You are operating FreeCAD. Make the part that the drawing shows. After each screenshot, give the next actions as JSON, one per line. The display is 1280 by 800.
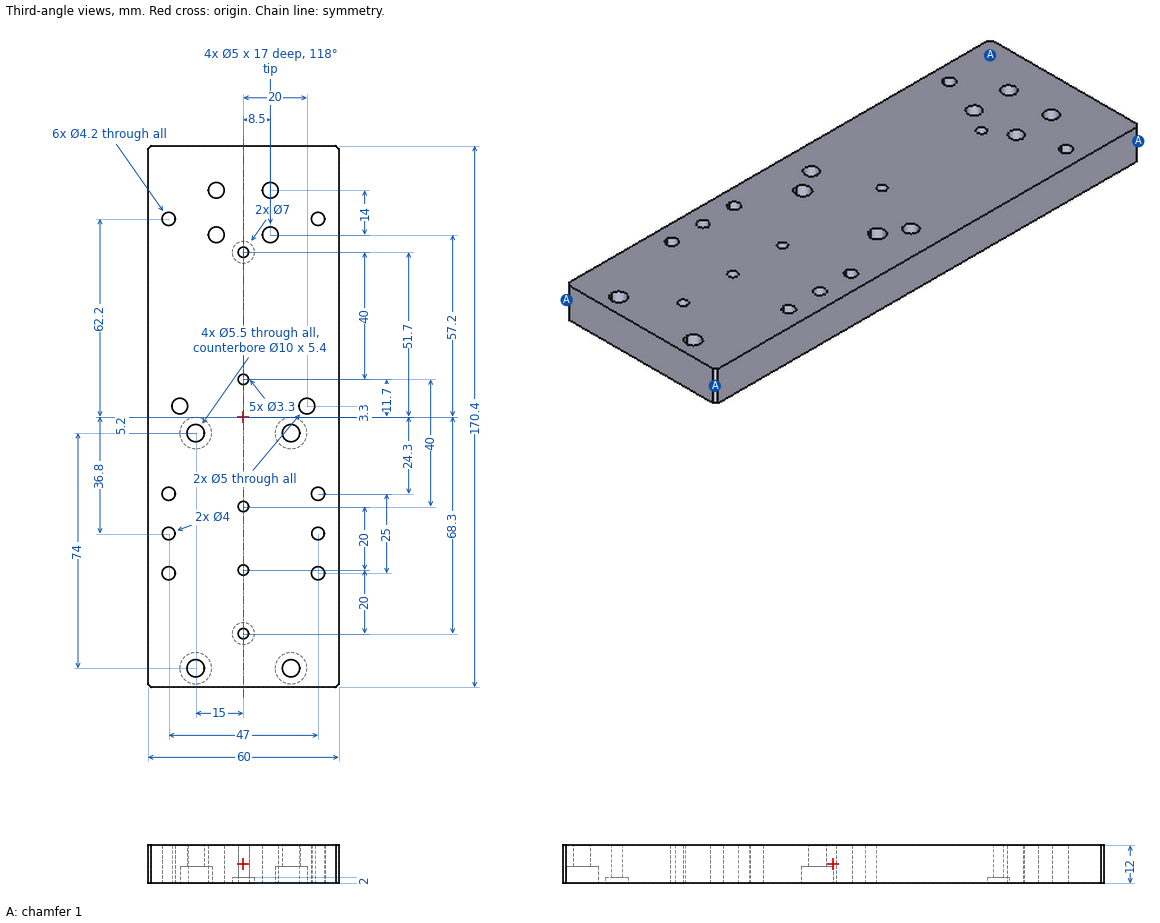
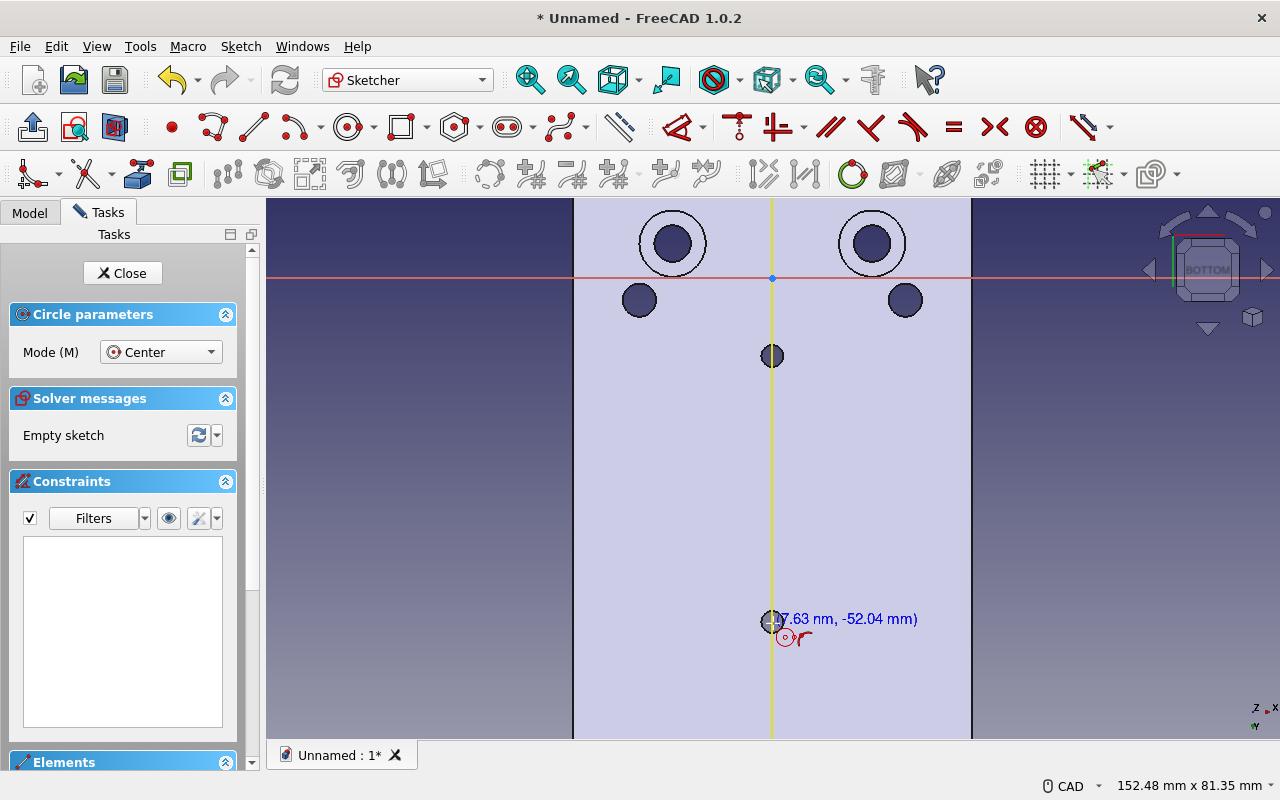
{"action": "left_click", "coordinate": [772, 622]}
{"action": "left_click", "coordinate": [789, 606]}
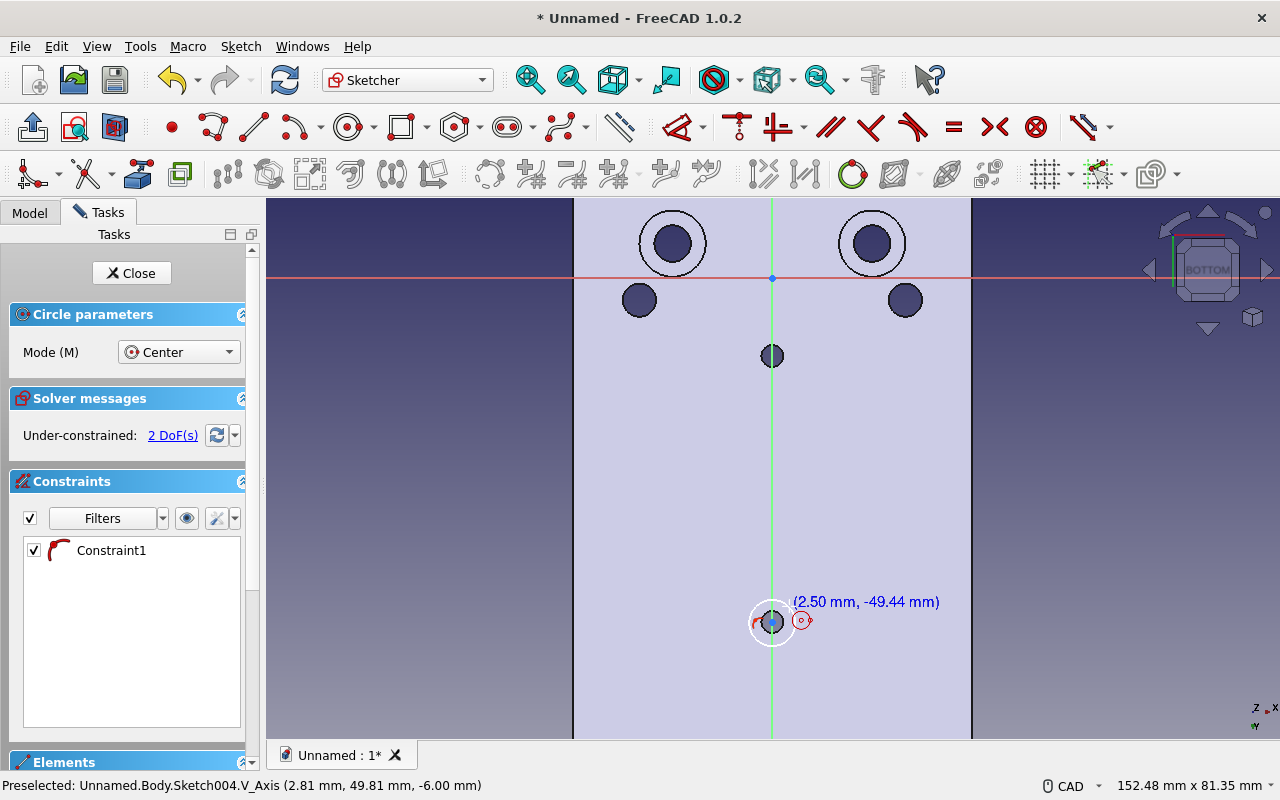
{"action": "scroll", "coordinate": [665, 611], "scroll_direction": "down", "scroll_amount": 5}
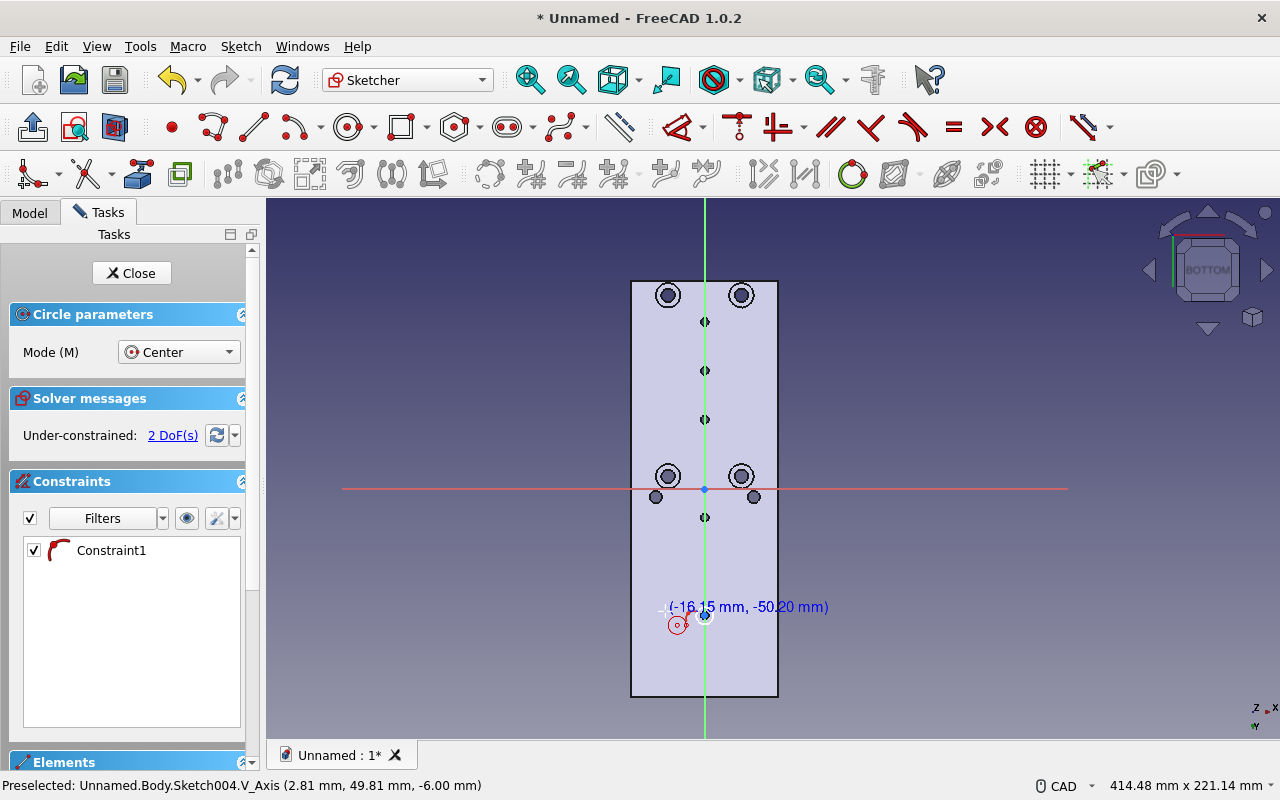
{"action": "scroll", "coordinate": [705, 322], "scroll_direction": "up", "scroll_amount": 5}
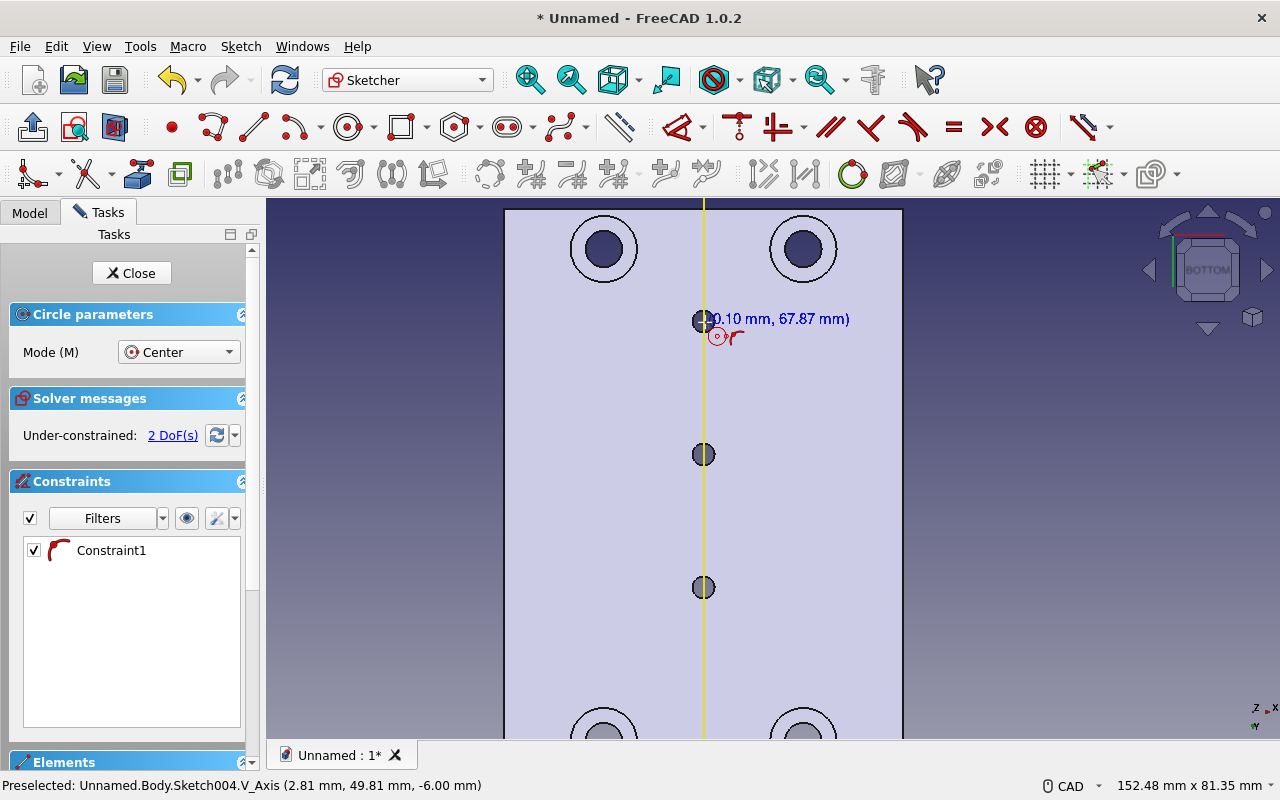
{"action": "left_click", "coordinate": [704, 321]}
{"action": "left_click", "coordinate": [720, 305]}
{"action": "key", "text": "Escape"}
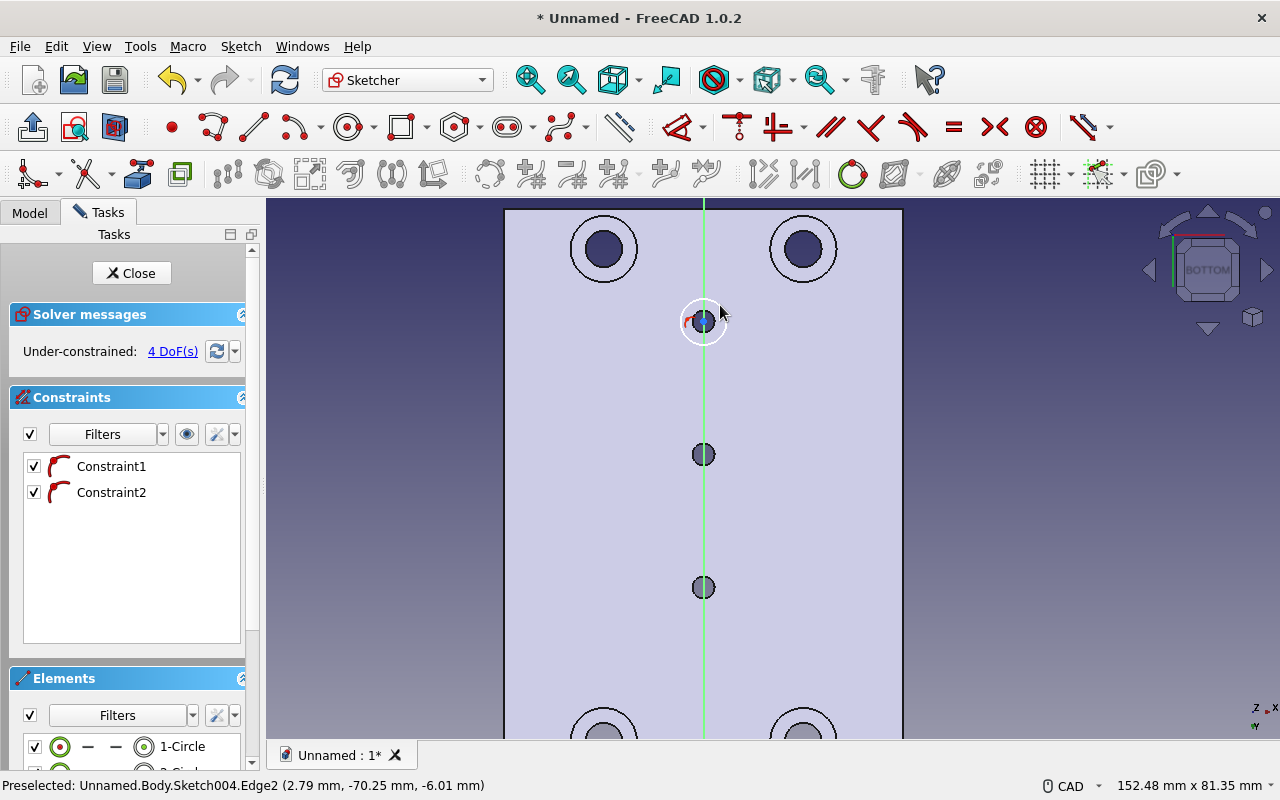
{"action": "scroll", "coordinate": [705, 322], "scroll_direction": "down", "scroll_amount": 5}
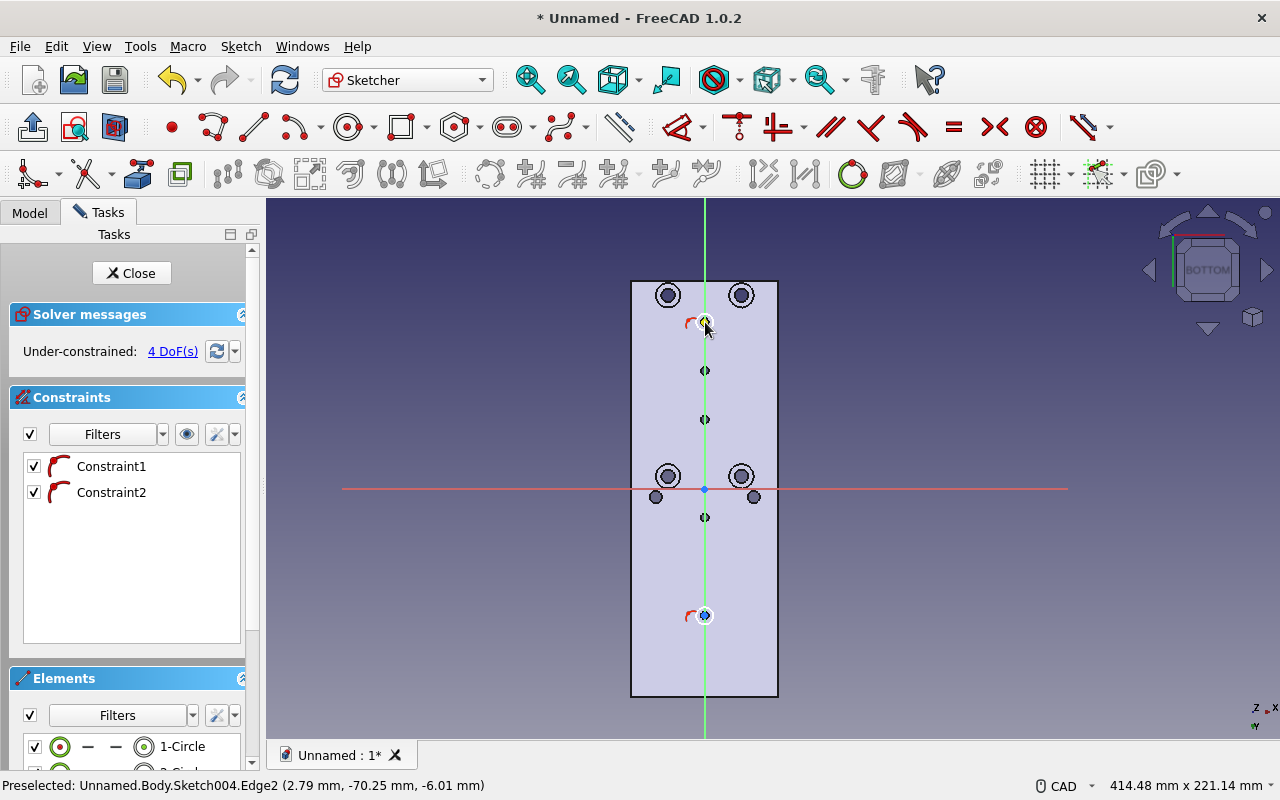
{"action": "scroll", "coordinate": [711, 610], "scroll_direction": "up", "scroll_amount": 5}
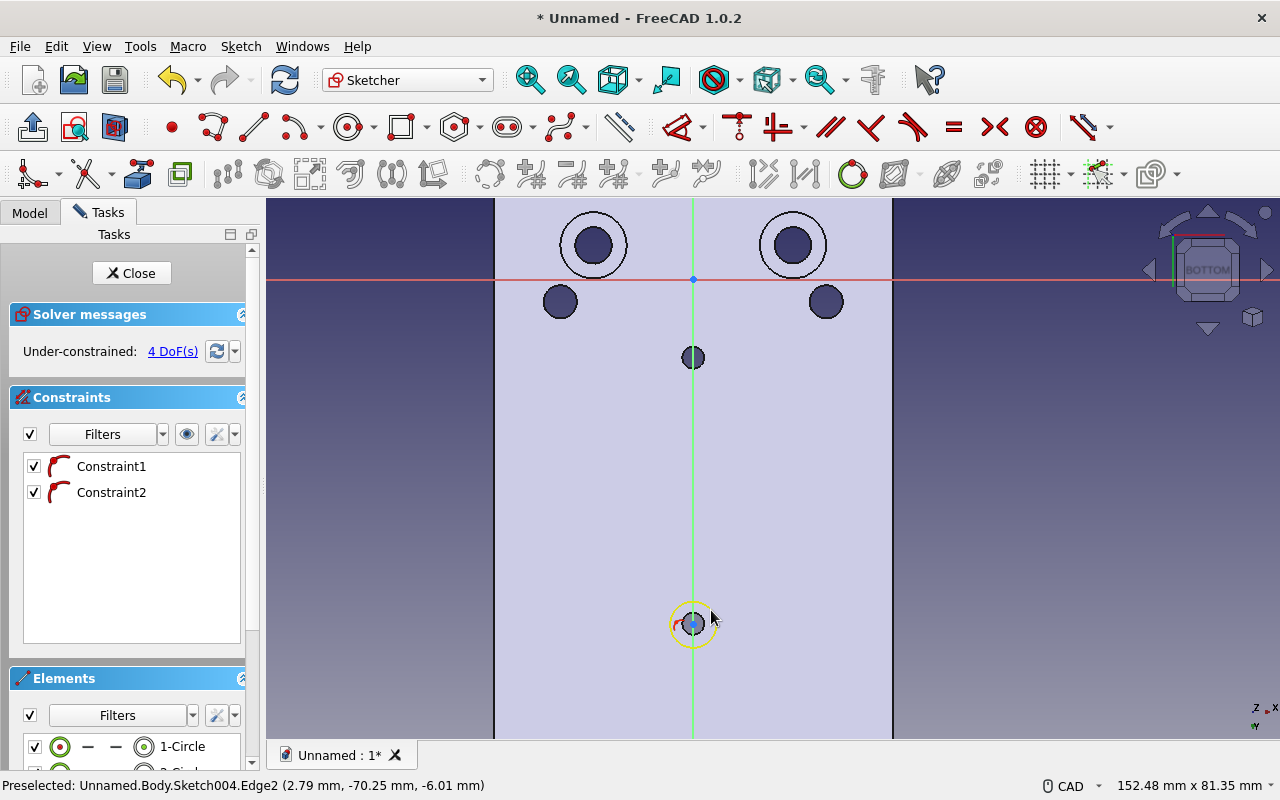
{"action": "left_click", "coordinate": [710, 608]}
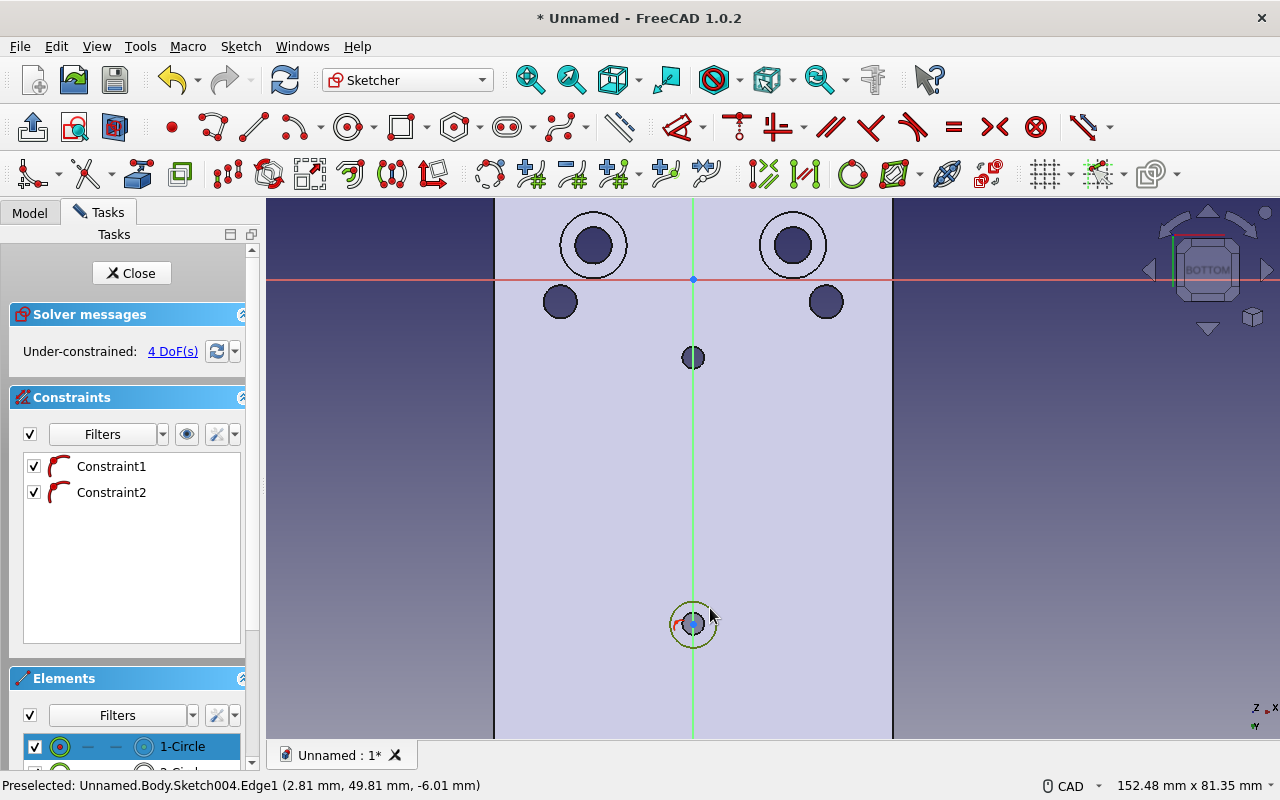
{"action": "scroll", "coordinate": [711, 610], "scroll_direction": "down", "scroll_amount": 5}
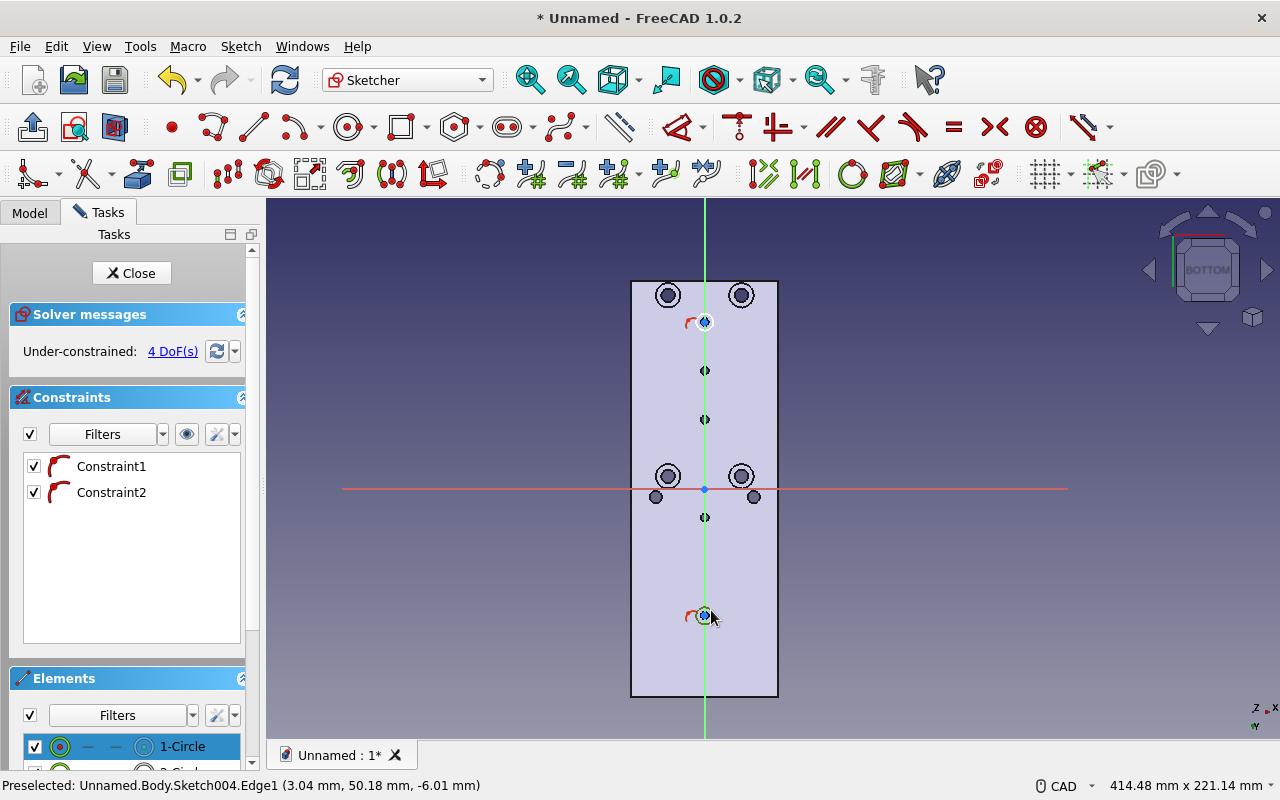
{"action": "scroll", "coordinate": [711, 316], "scroll_direction": "up", "scroll_amount": 5}